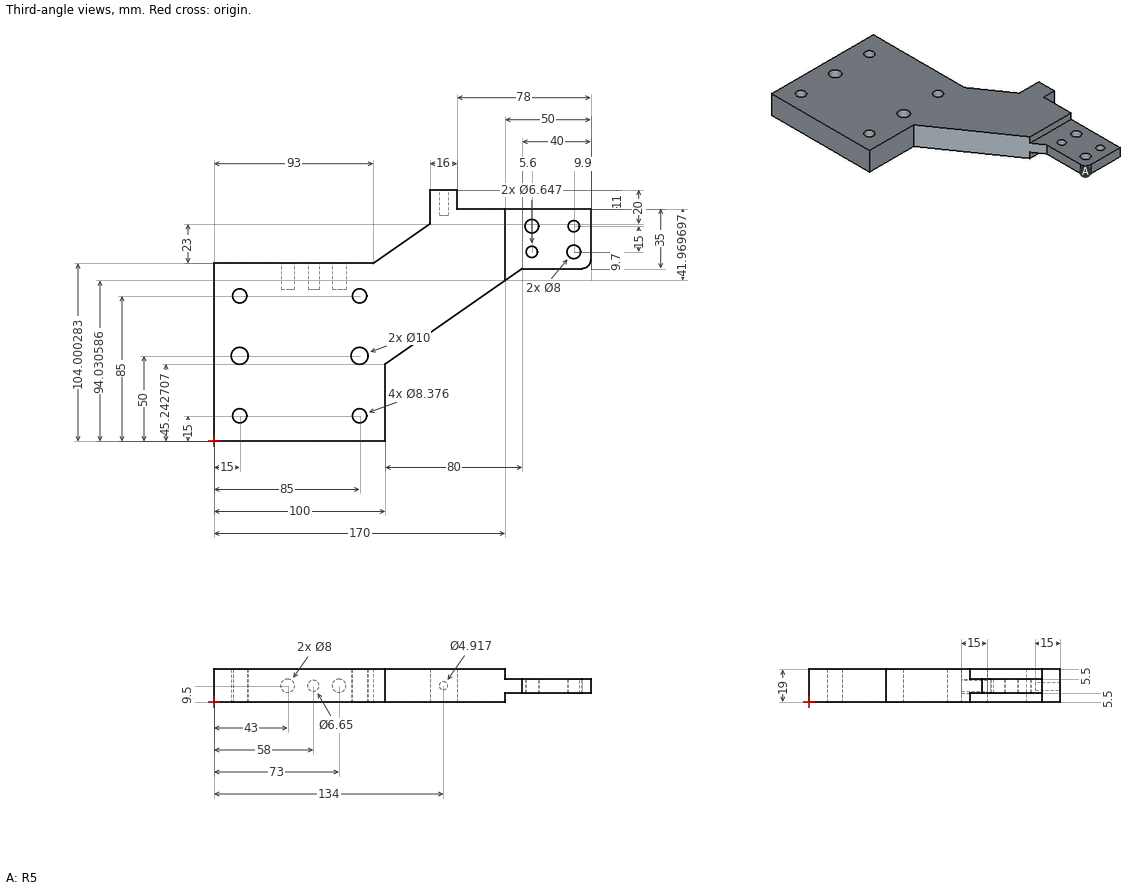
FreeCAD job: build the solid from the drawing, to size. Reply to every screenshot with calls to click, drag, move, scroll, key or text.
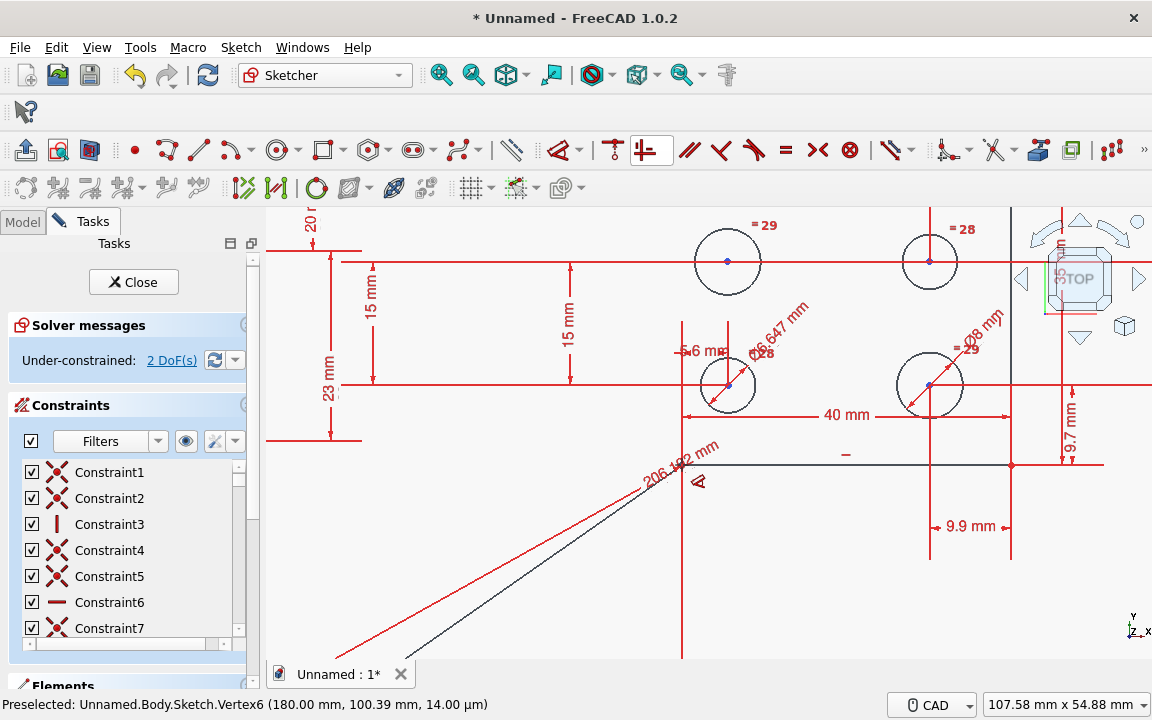
click(728, 262)
click(705, 499)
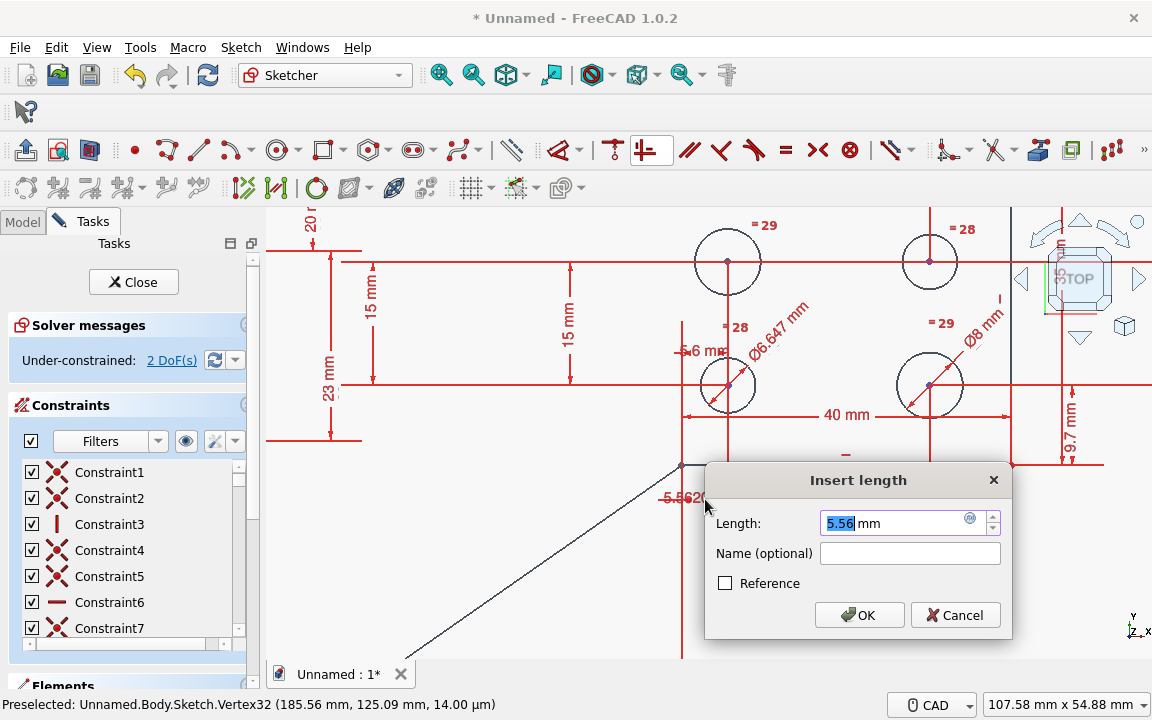
text(5.6)
key(Return)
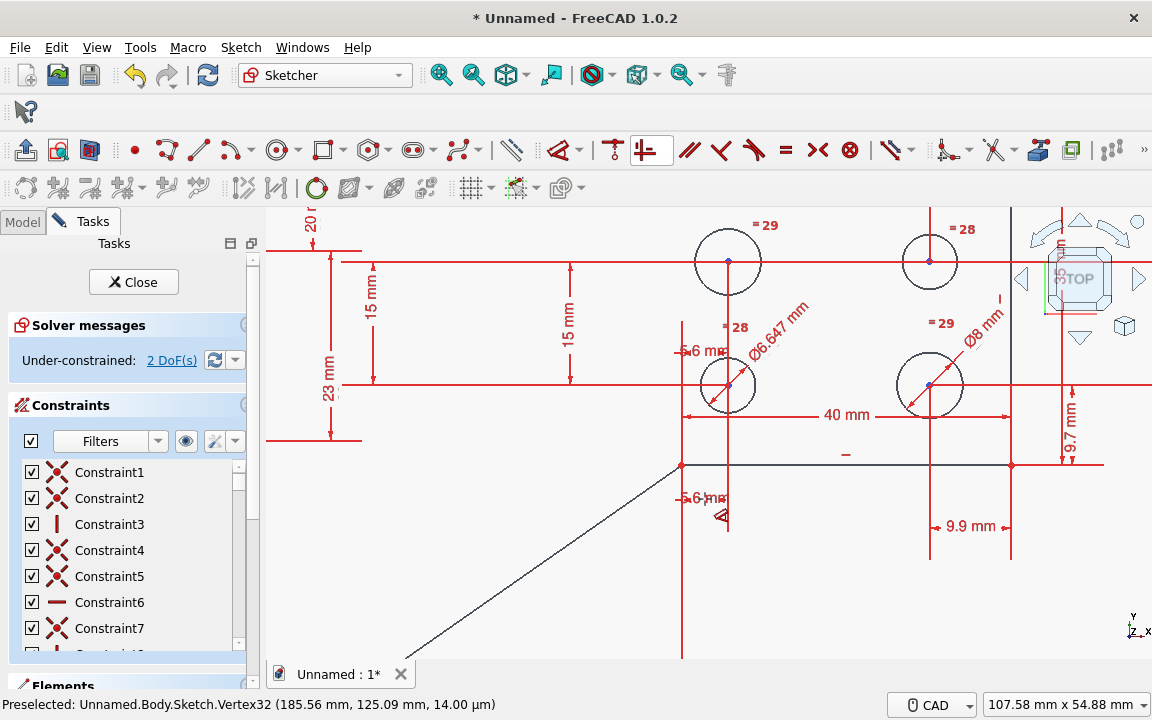
scroll(816, 350, down, 7)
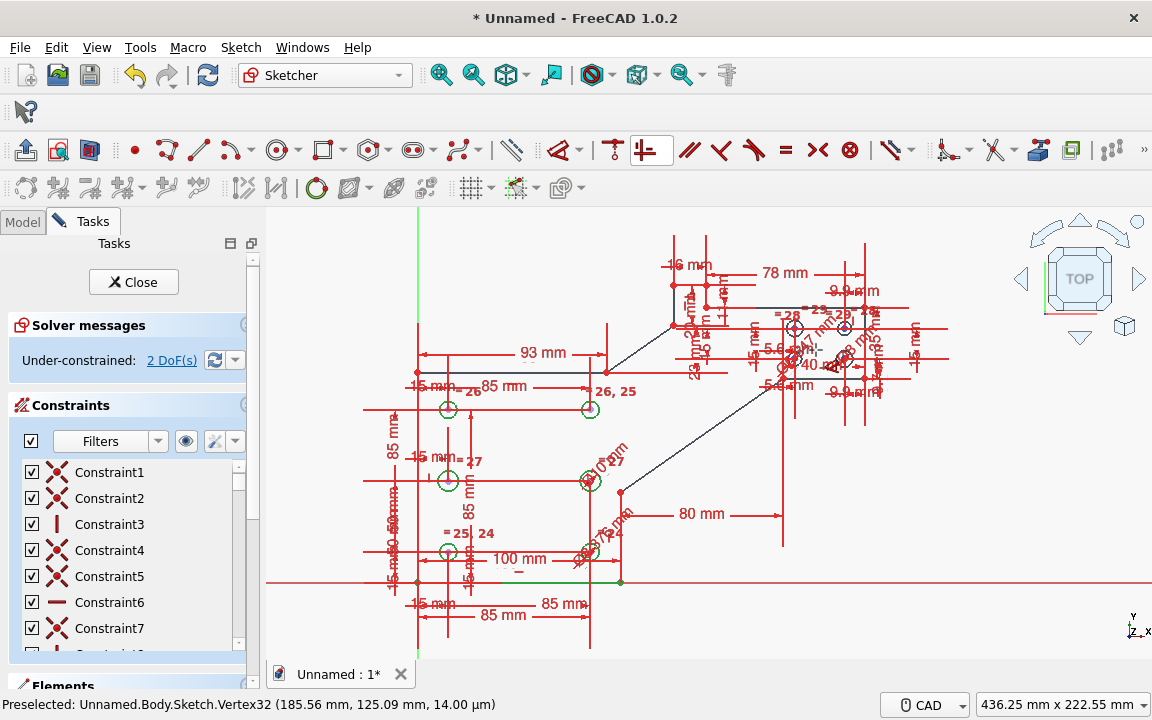
click(621, 556)
click(587, 517)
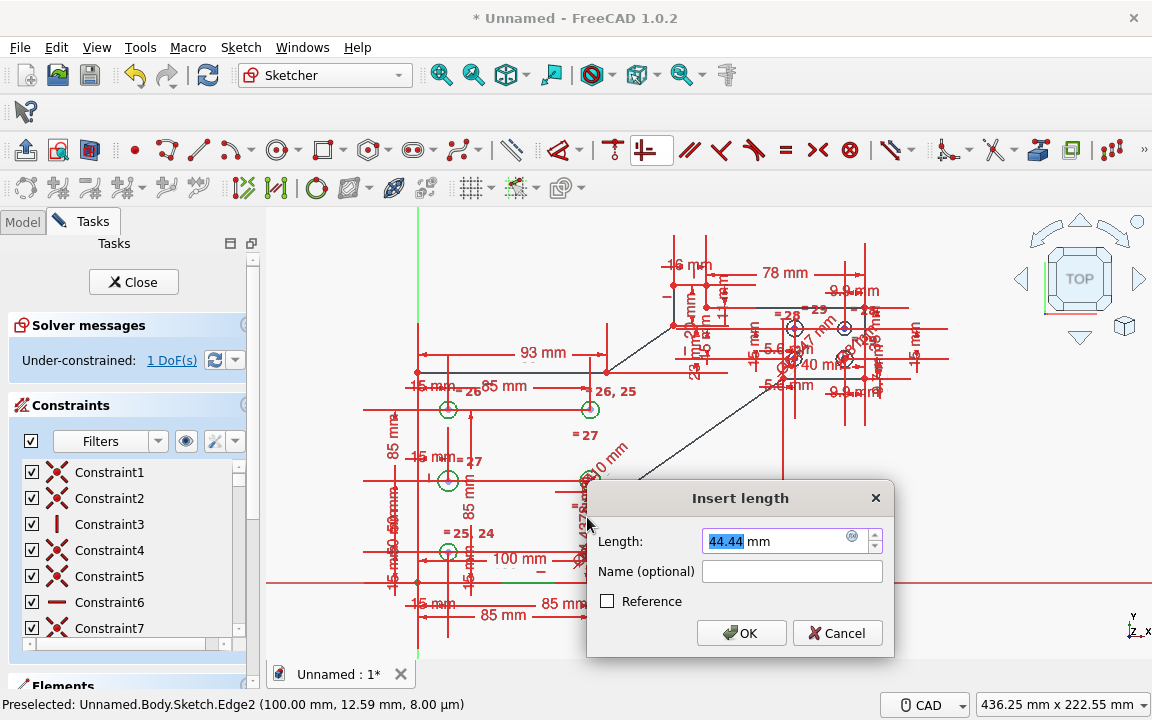
text(45.242707)
key(Return)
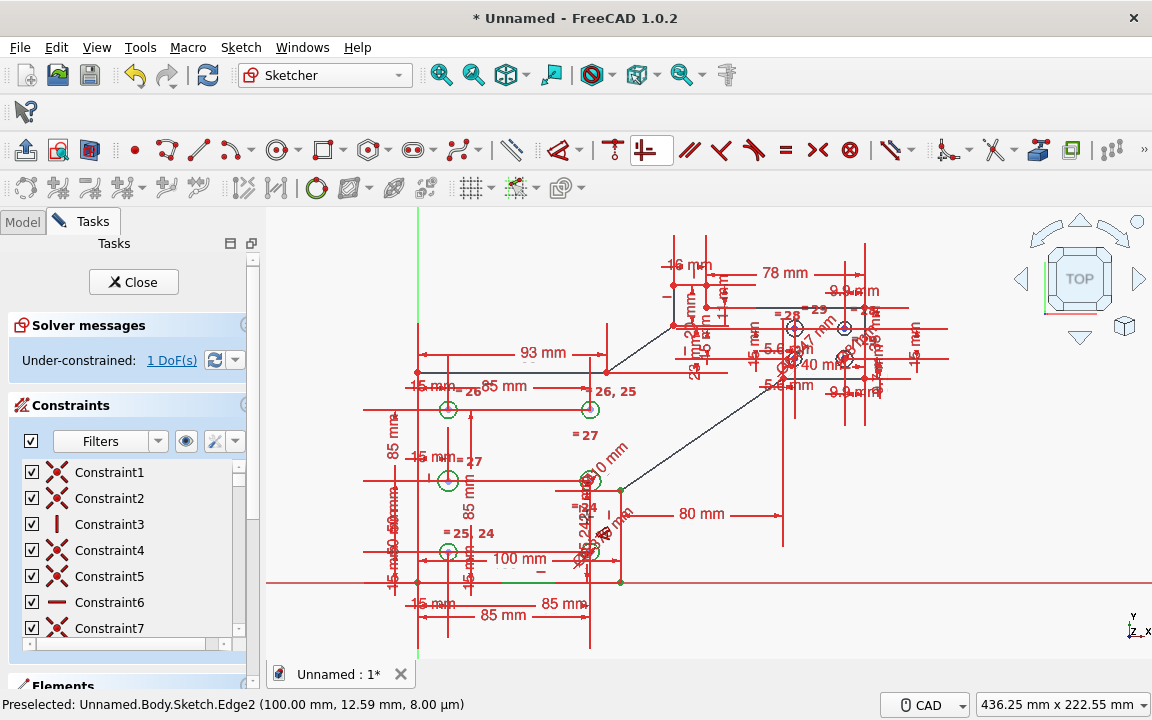
click(418, 436)
click(360, 478)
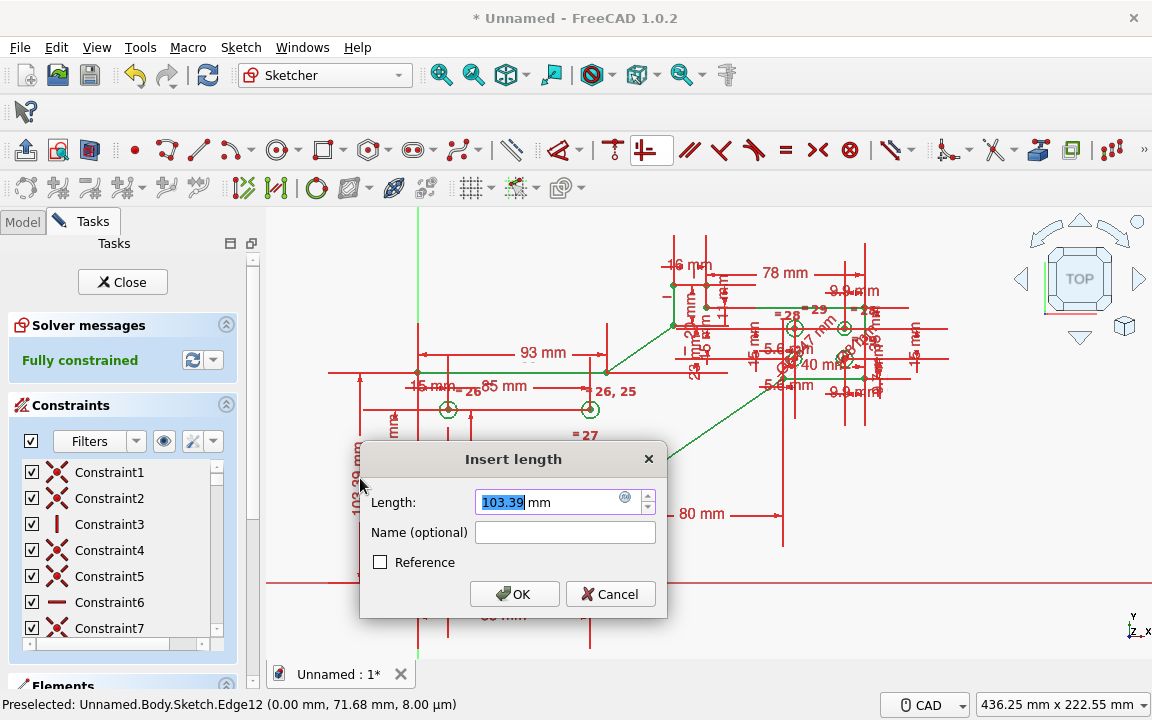
text(104.000283)
key(Return)
key(Escape)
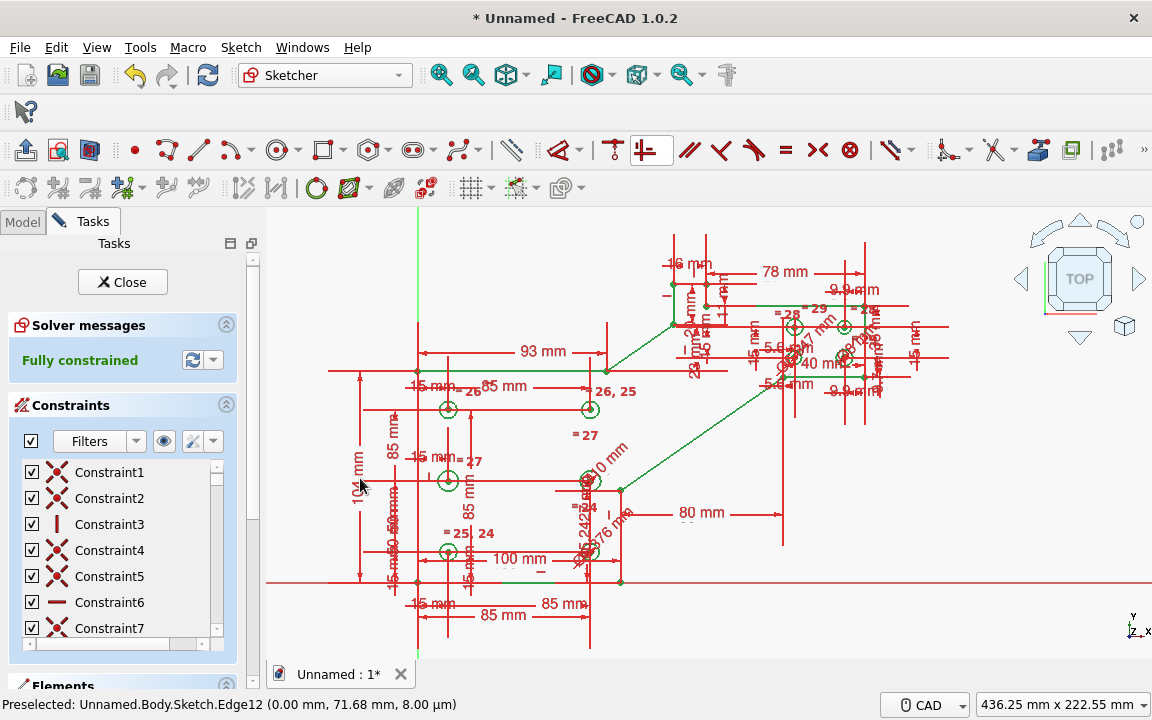
click(123, 282)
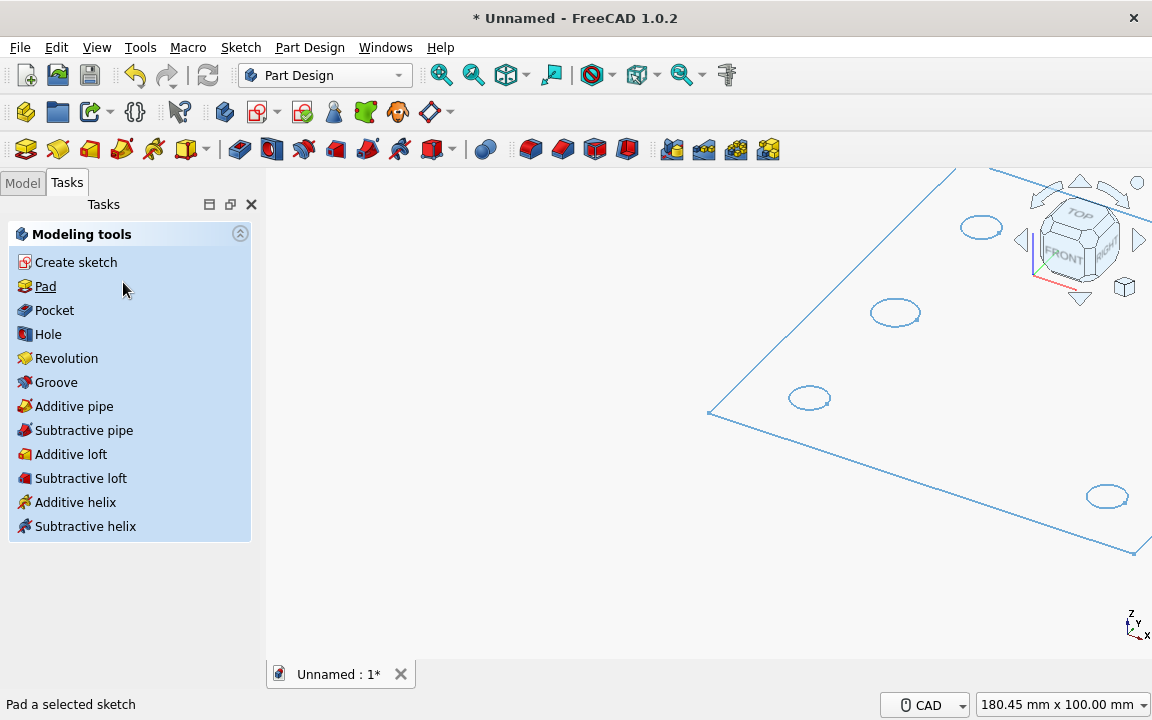
click(26, 150)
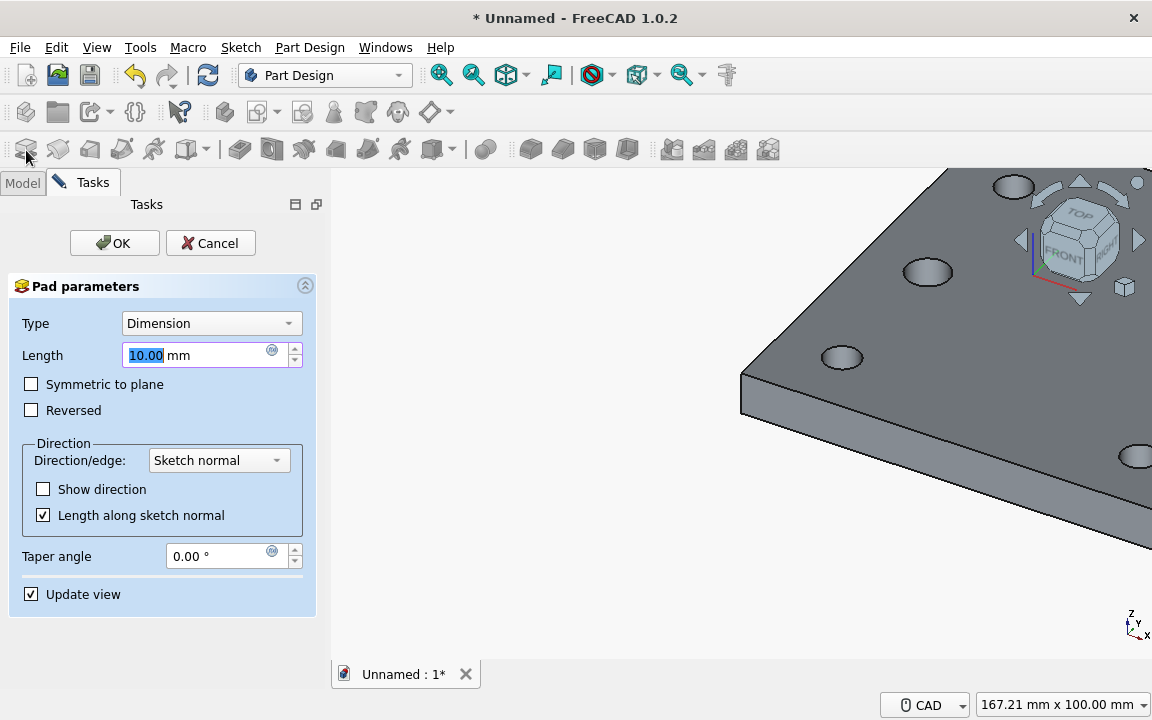
text(19)
key(Tab)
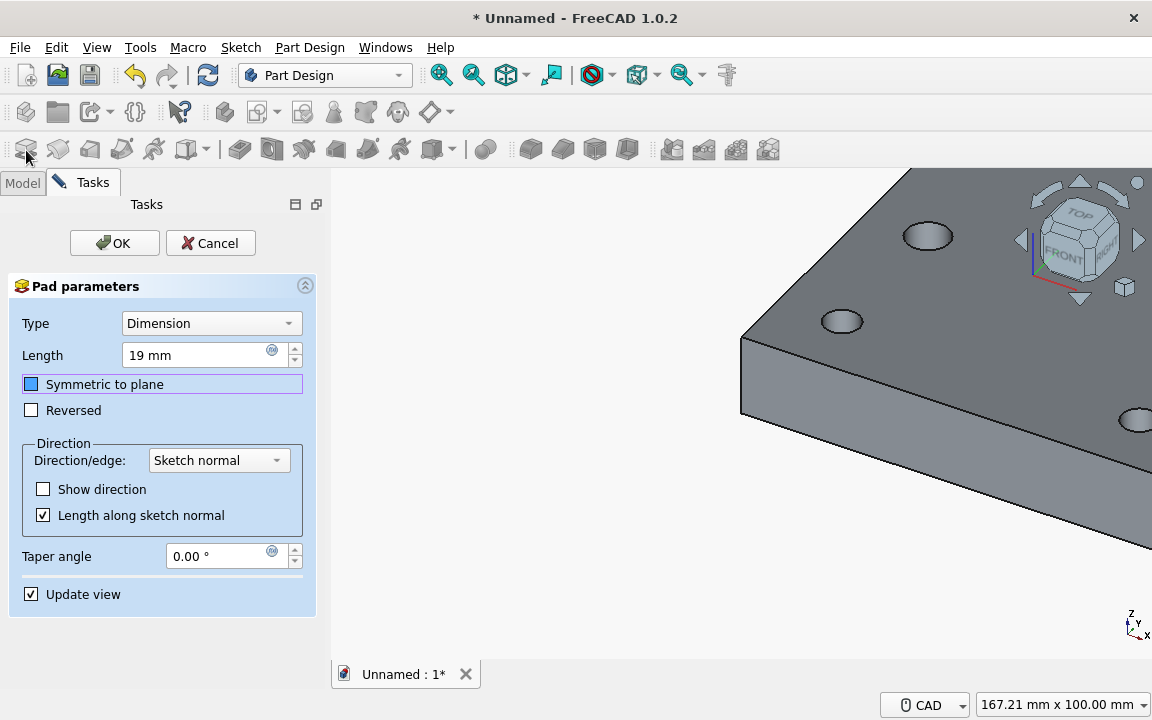
click(115, 243)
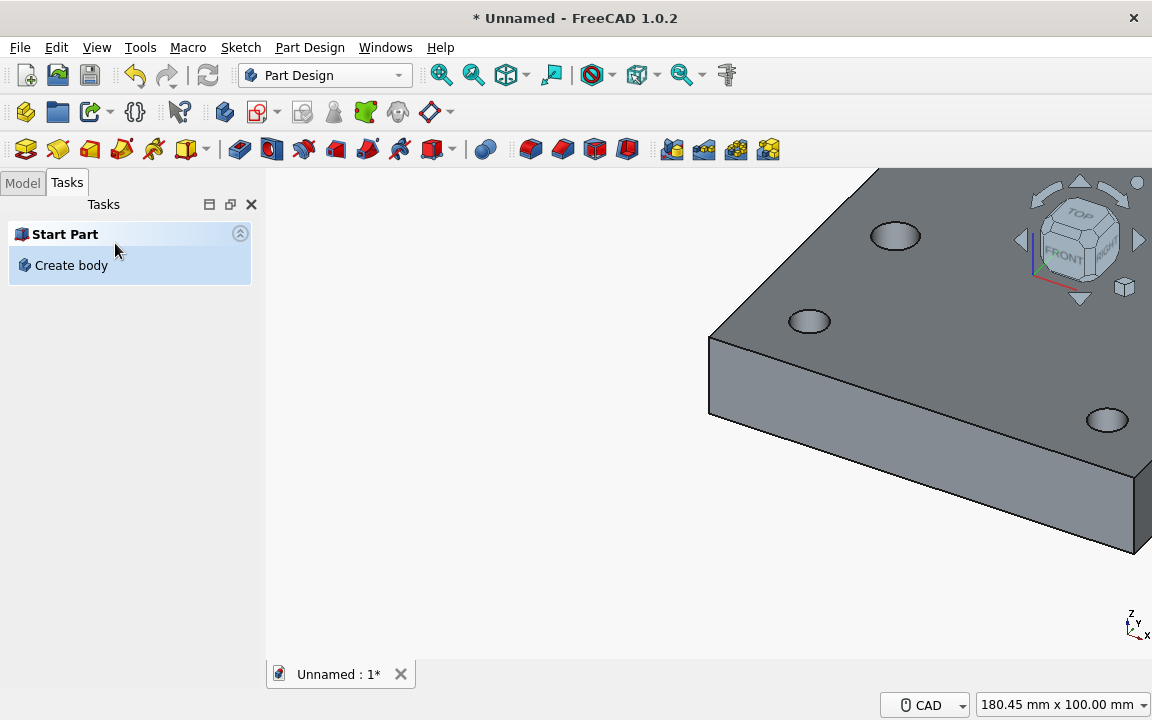
click(442, 76)